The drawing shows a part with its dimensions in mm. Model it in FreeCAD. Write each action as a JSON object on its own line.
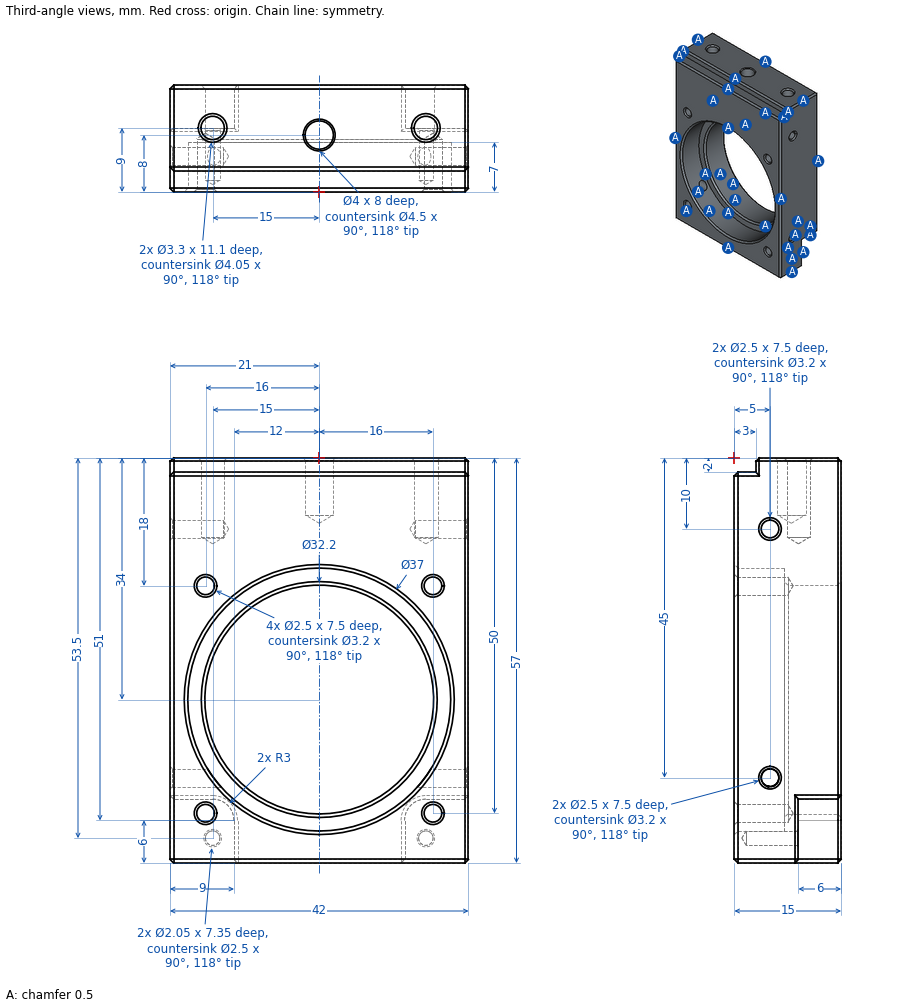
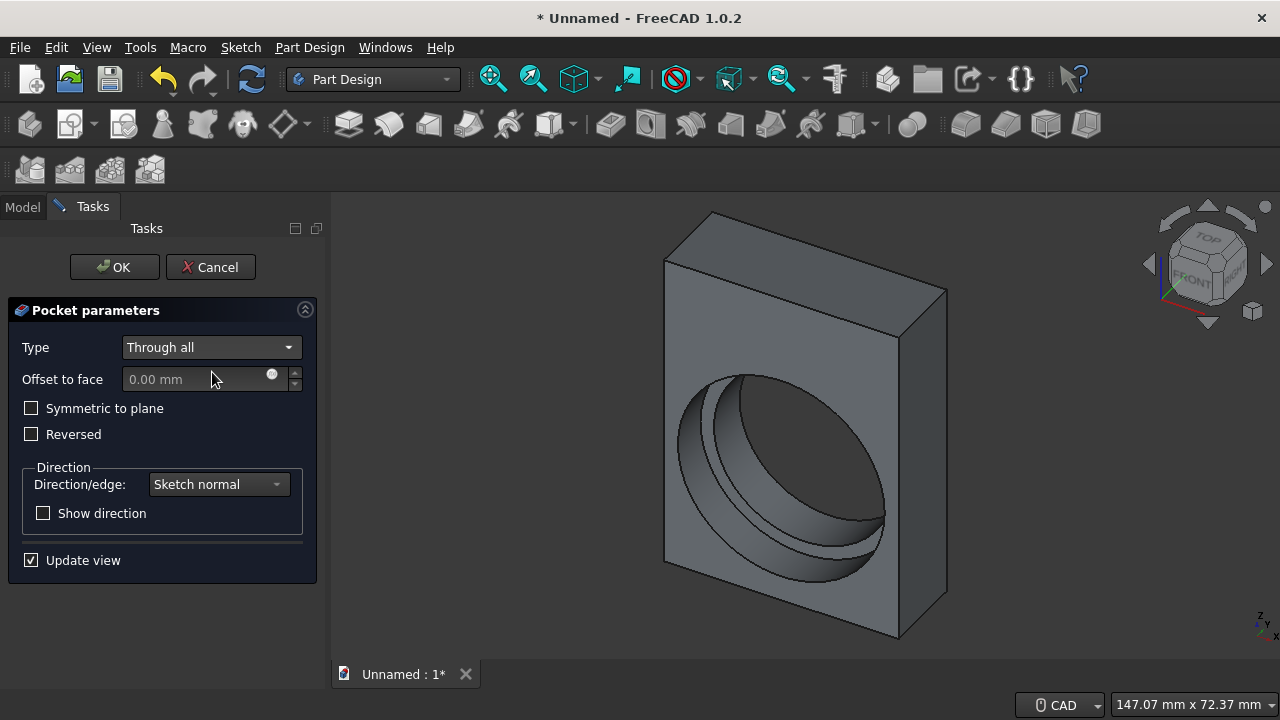
{"action": "left_click", "coordinate": [115, 267]}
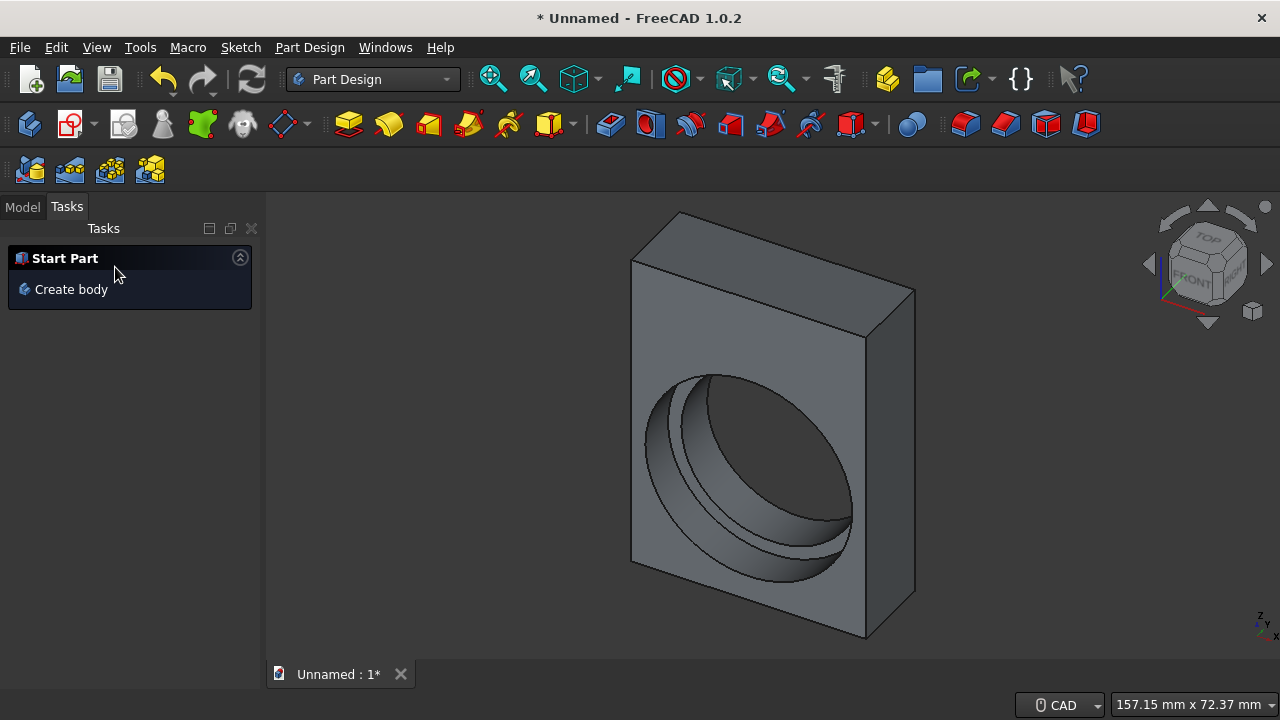
{"action": "left_click", "coordinate": [890, 377]}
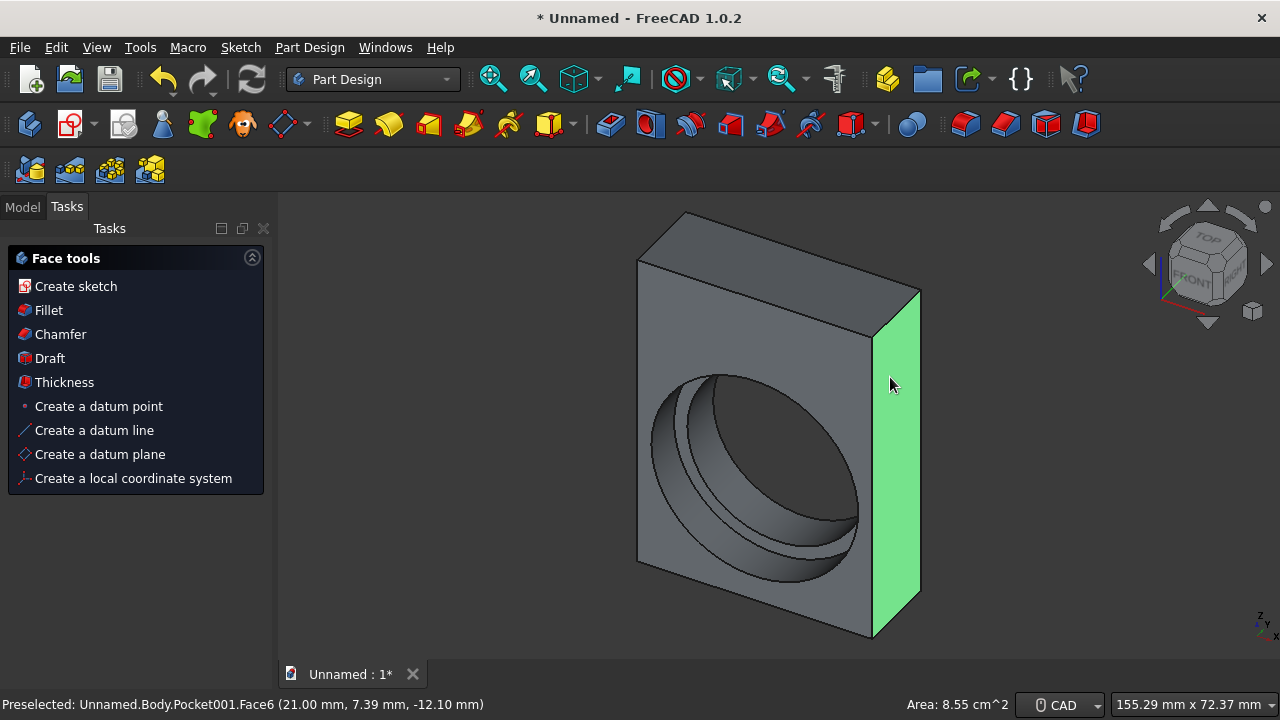
{"action": "left_click", "coordinate": [70, 124]}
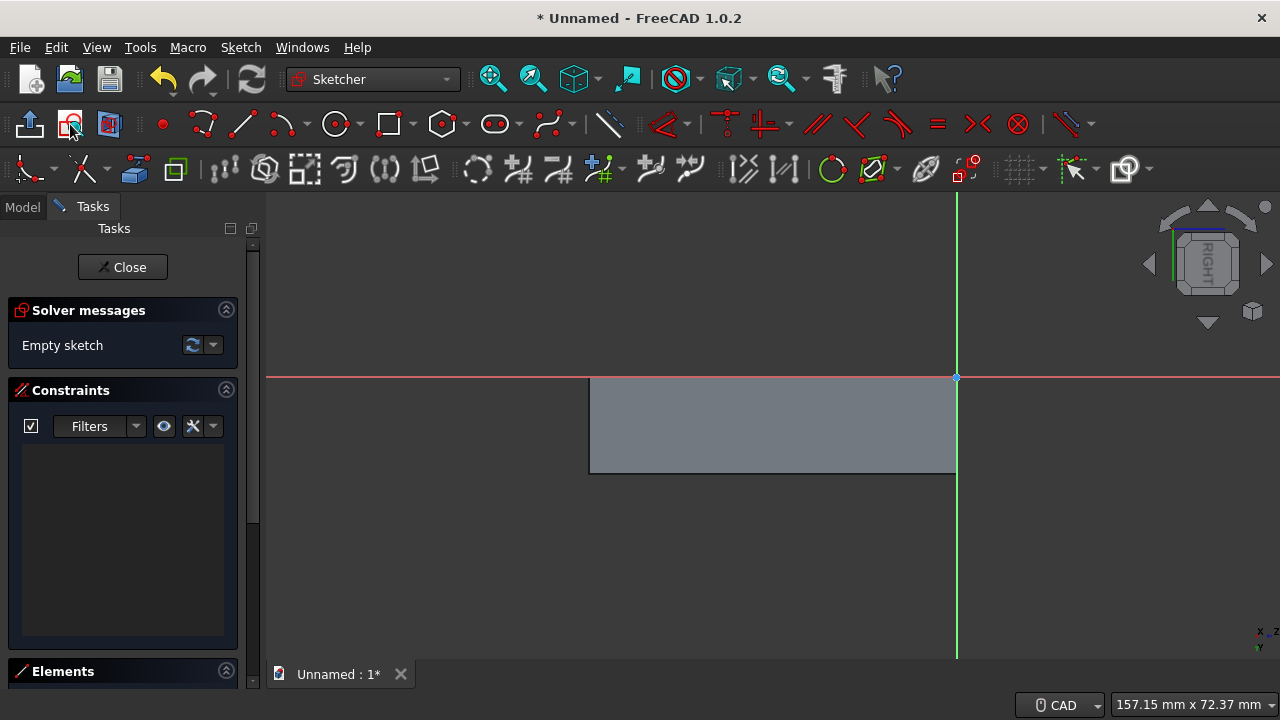
{"action": "scroll", "coordinate": [966, 384], "scroll_direction": "up", "scroll_amount": 14}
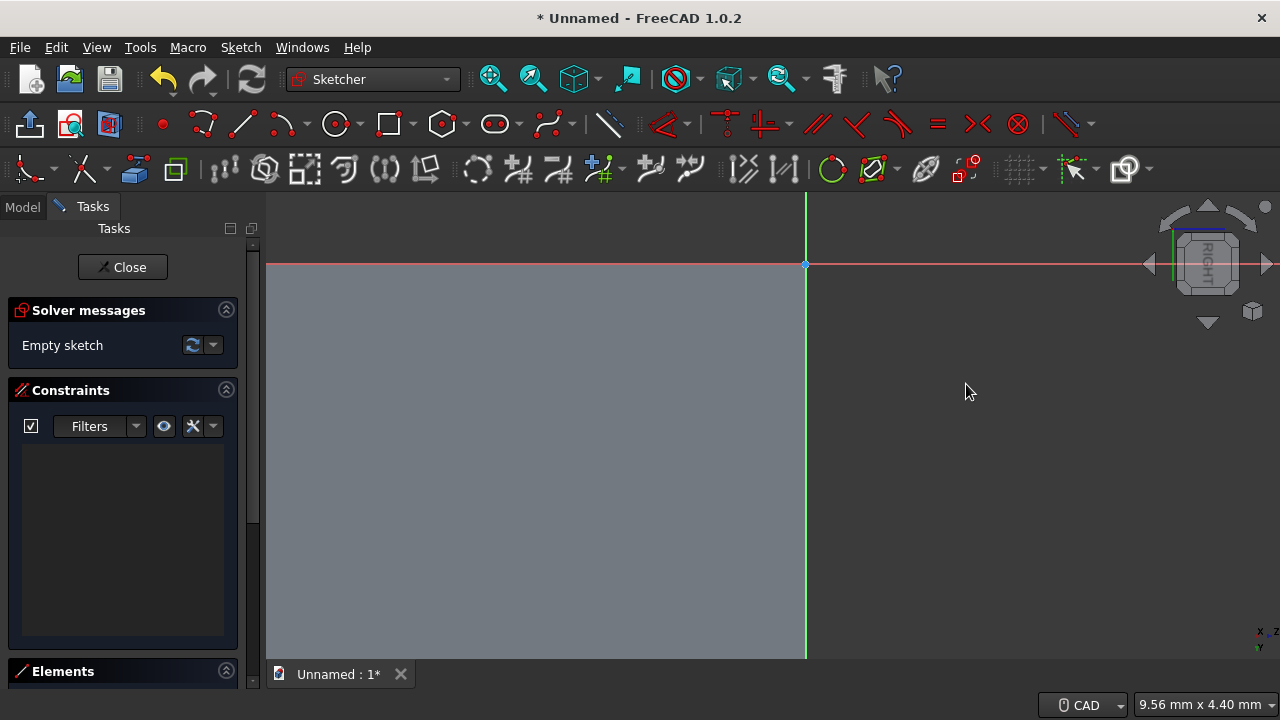
{"action": "key", "text": "g r"}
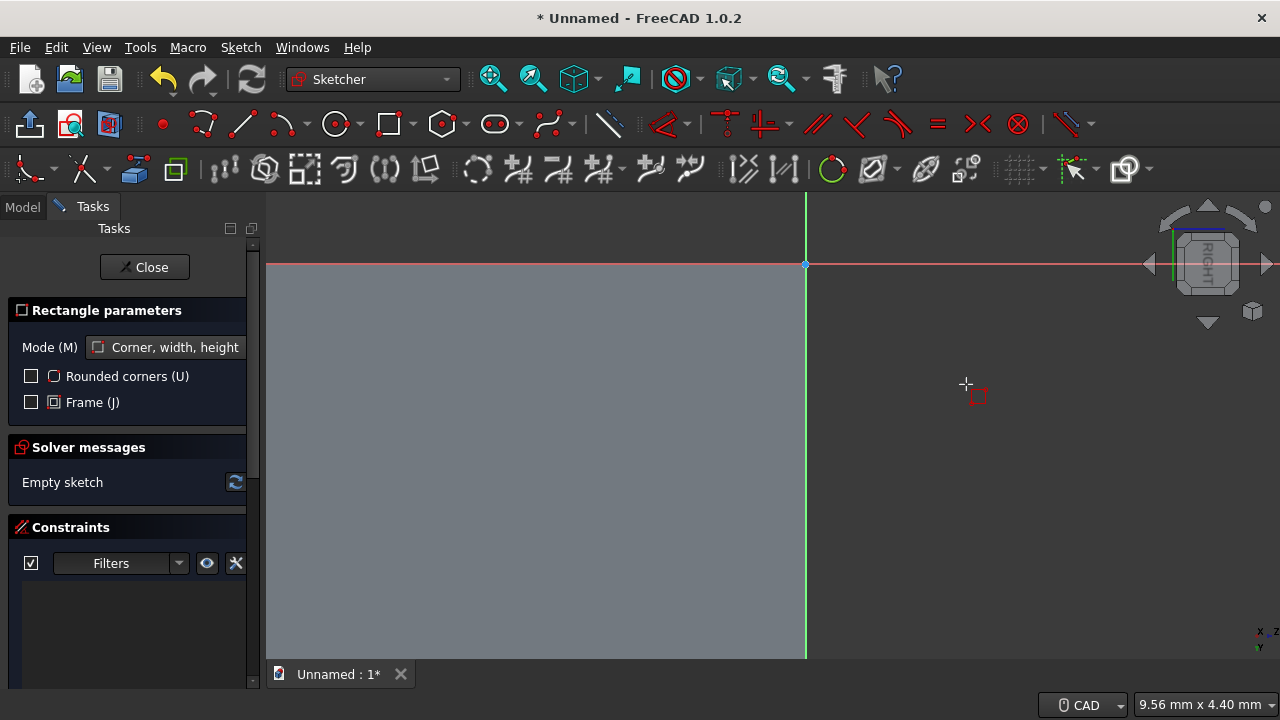
{"action": "left_click", "coordinate": [806, 264]}
{"action": "mouse_move", "coordinate": [593, 583]}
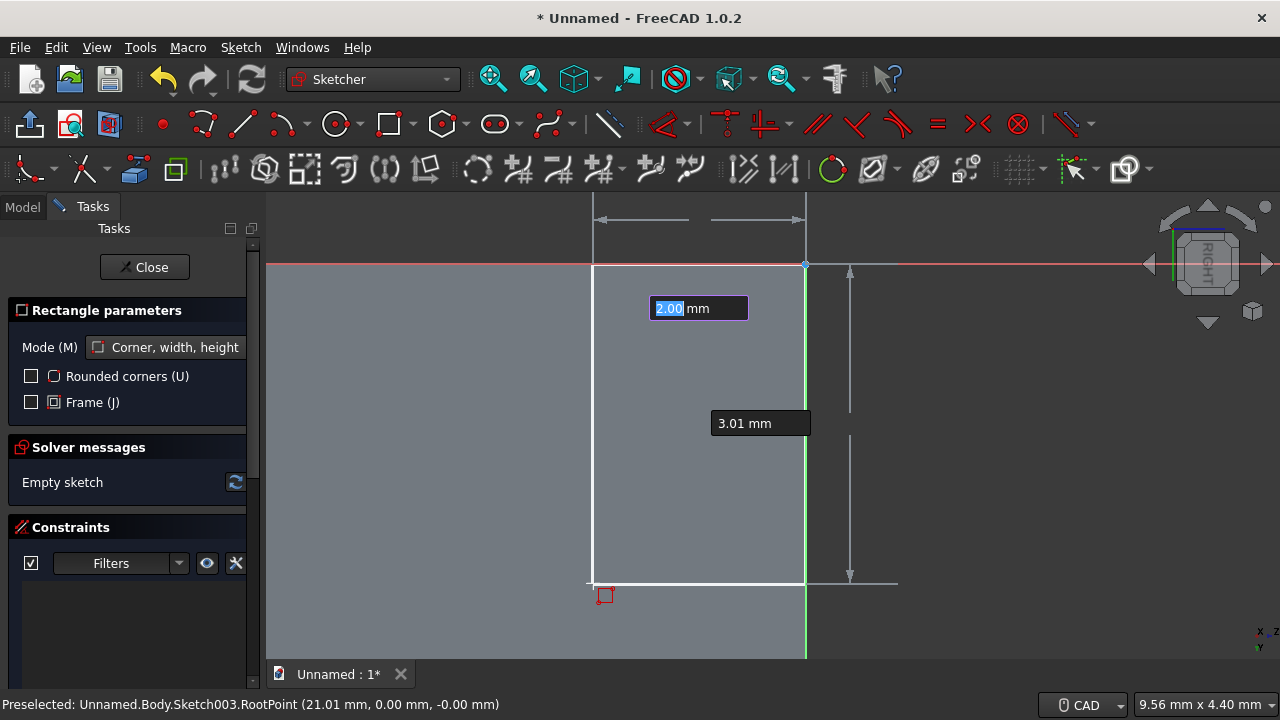
{"action": "type", "text": "2"}
{"action": "key", "text": "Tab"}
{"action": "type", "text": "3"}
{"action": "key", "text": "Return"}
{"action": "key", "text": "Escape"}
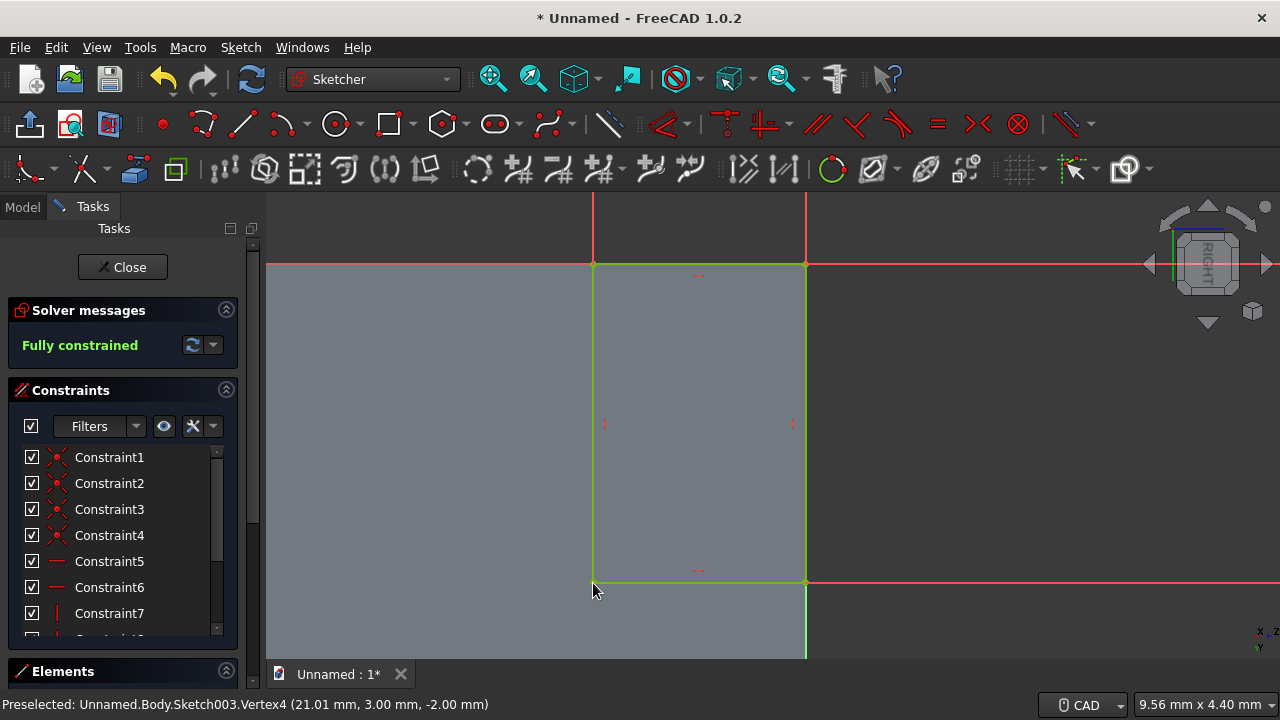
{"action": "left_click", "coordinate": [123, 267]}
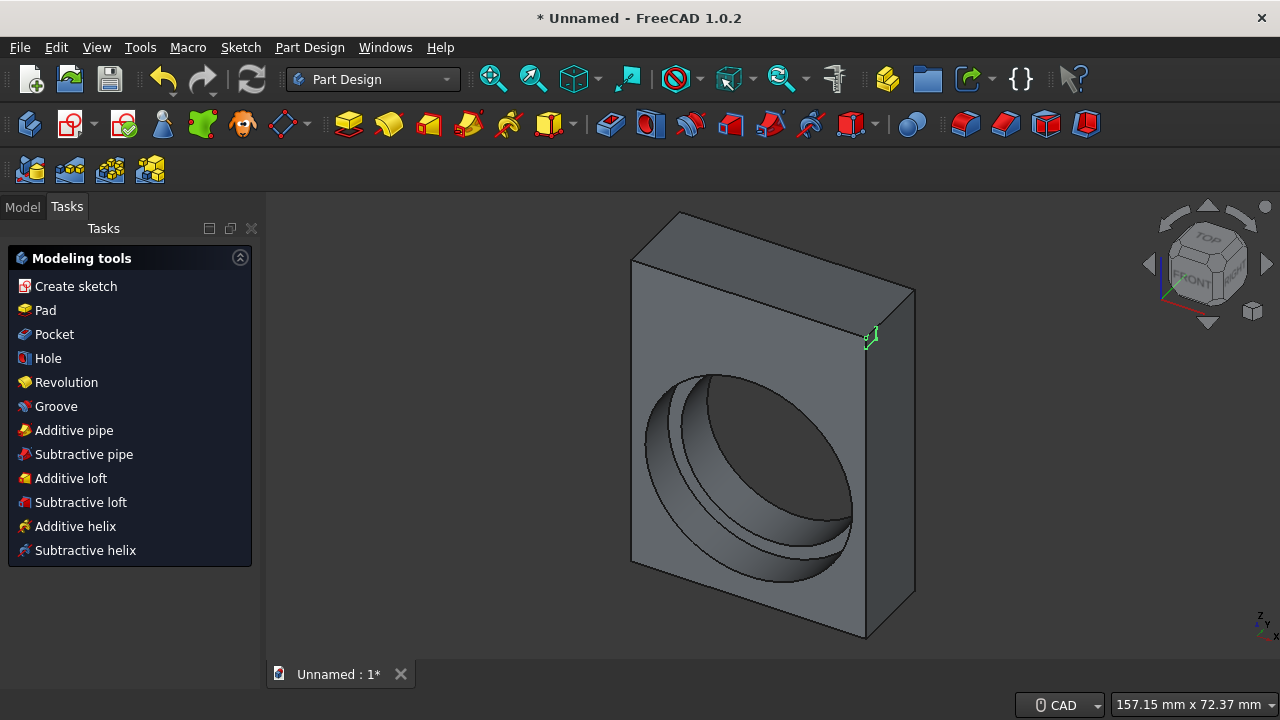
{"action": "left_click", "coordinate": [612, 124]}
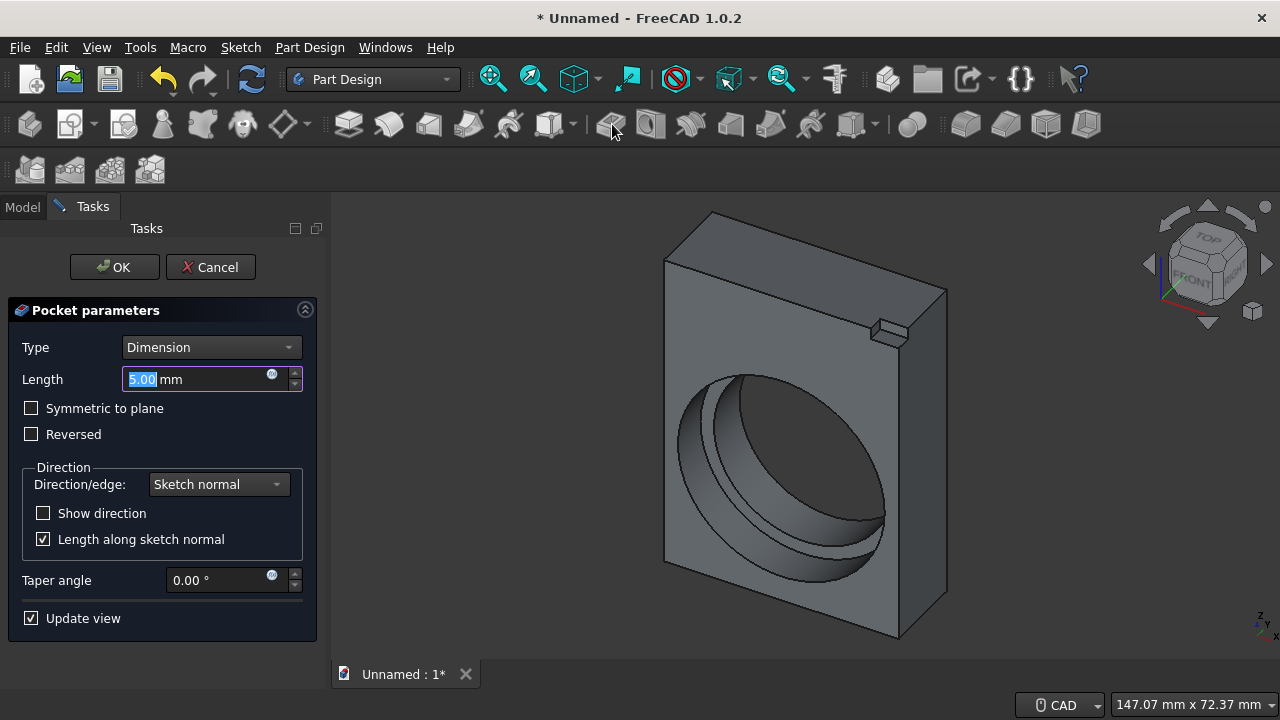
{"action": "left_click", "coordinate": [212, 348]}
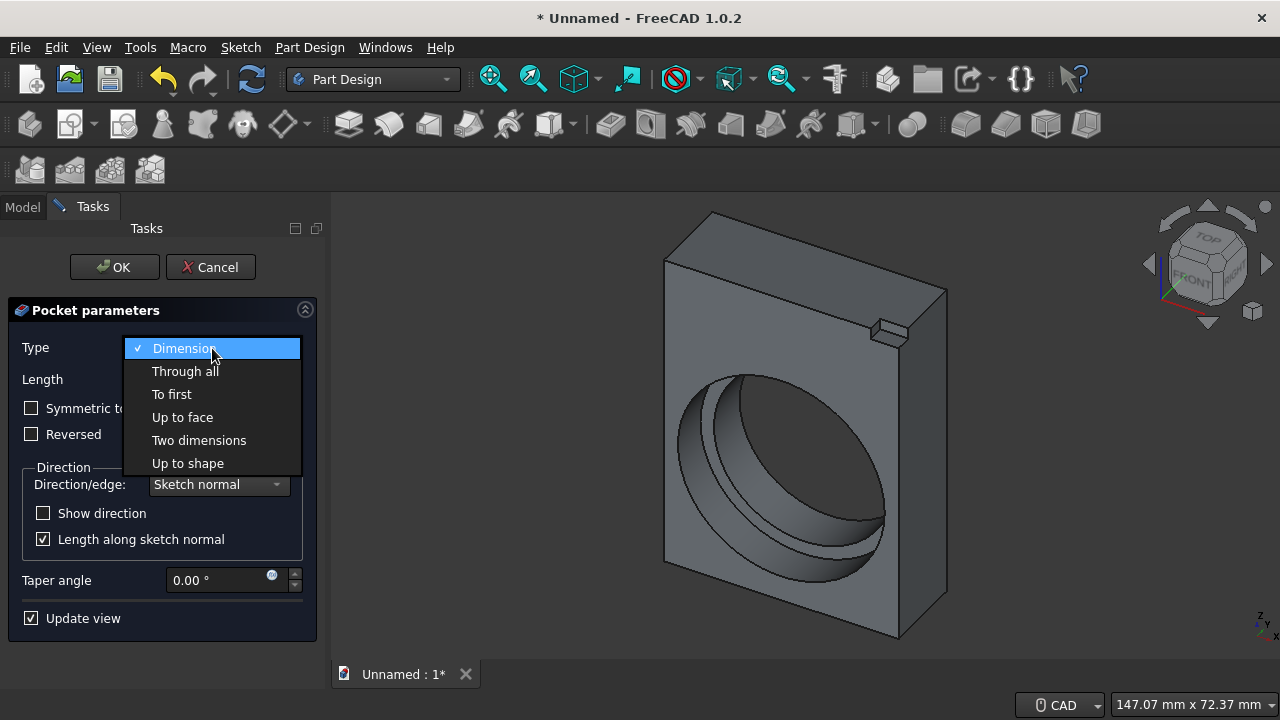
{"action": "left_click", "coordinate": [212, 372]}